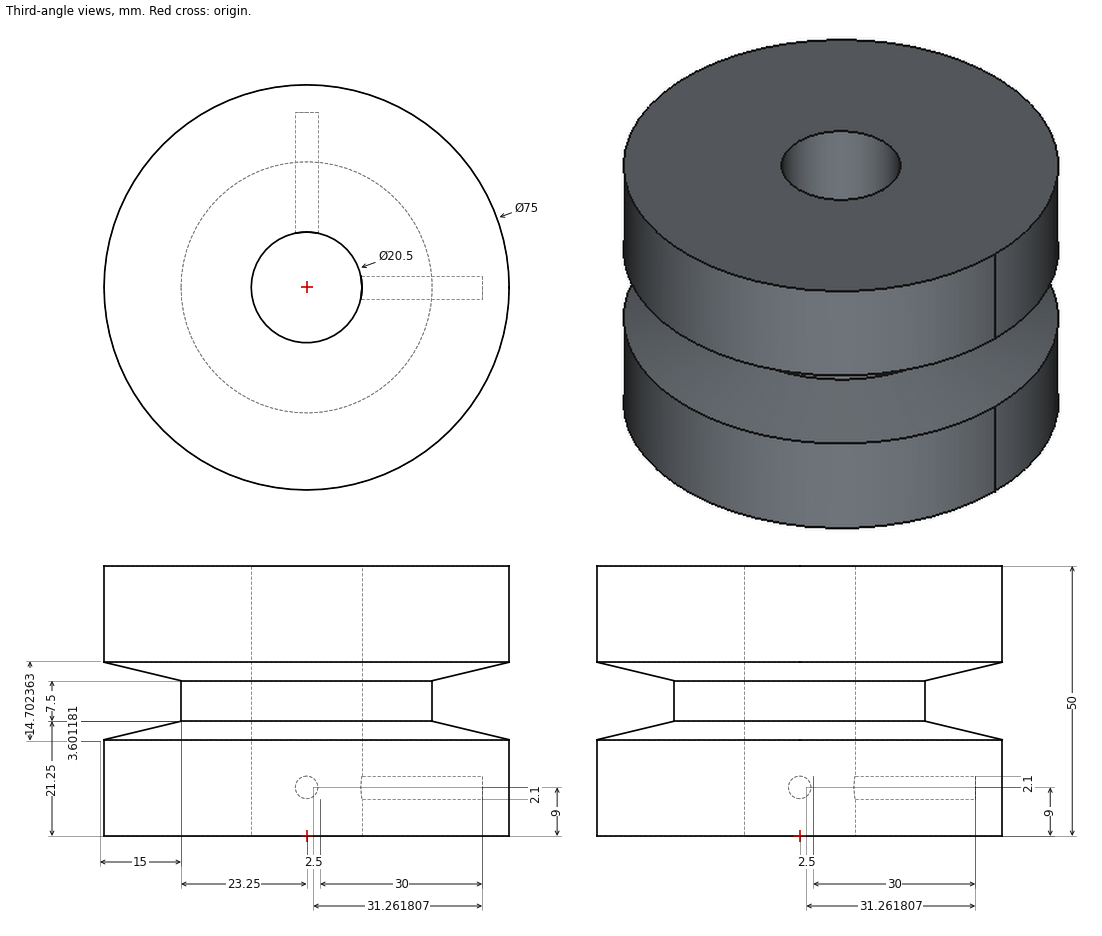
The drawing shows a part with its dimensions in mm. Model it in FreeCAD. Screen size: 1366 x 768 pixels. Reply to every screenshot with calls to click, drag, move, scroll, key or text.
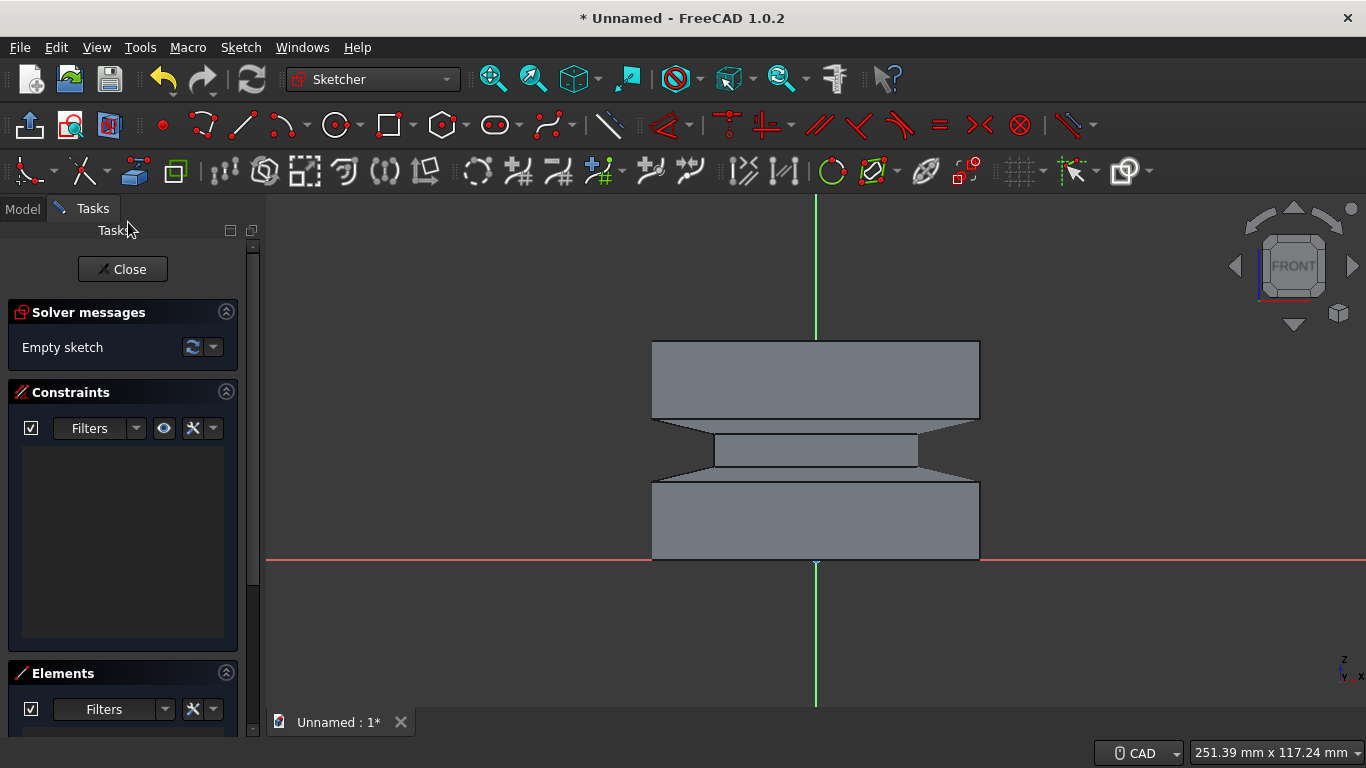
key(q)
key(s)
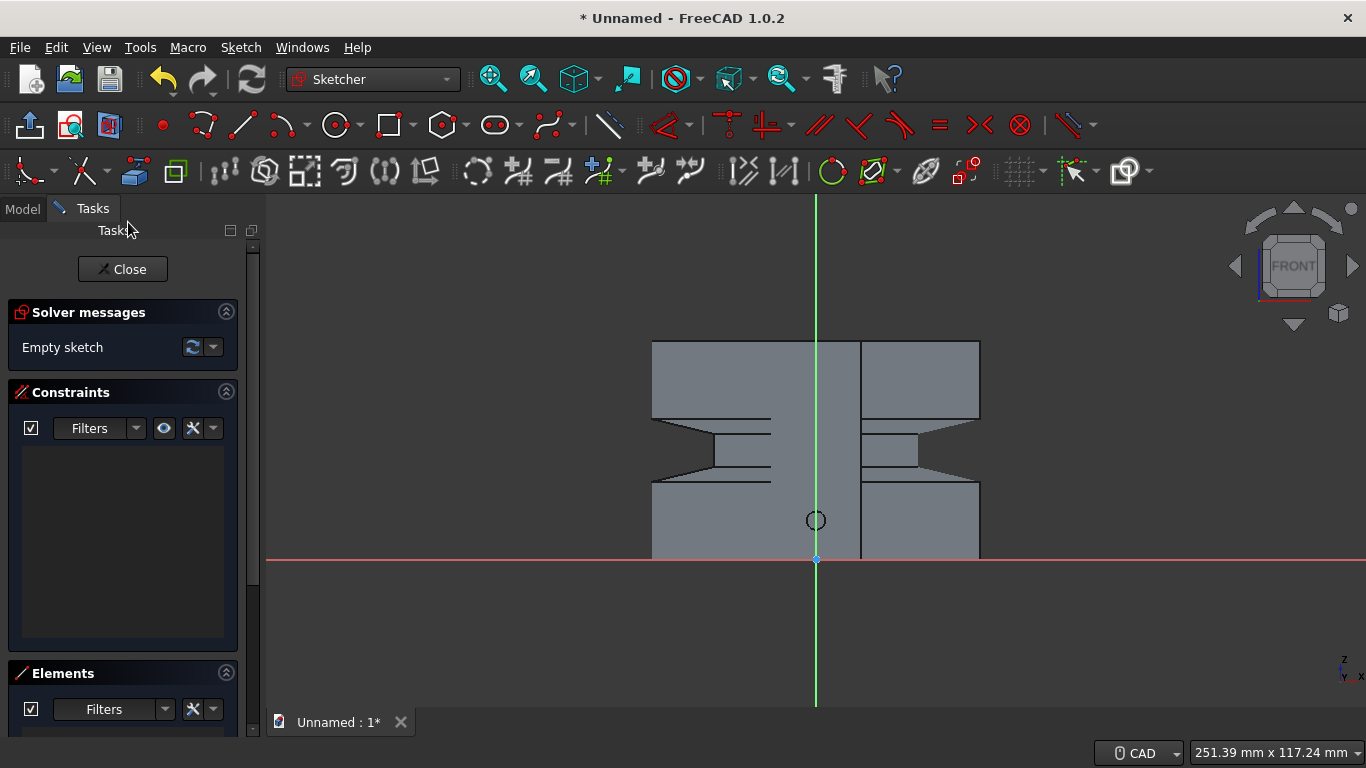
scroll(912, 579, up, 6)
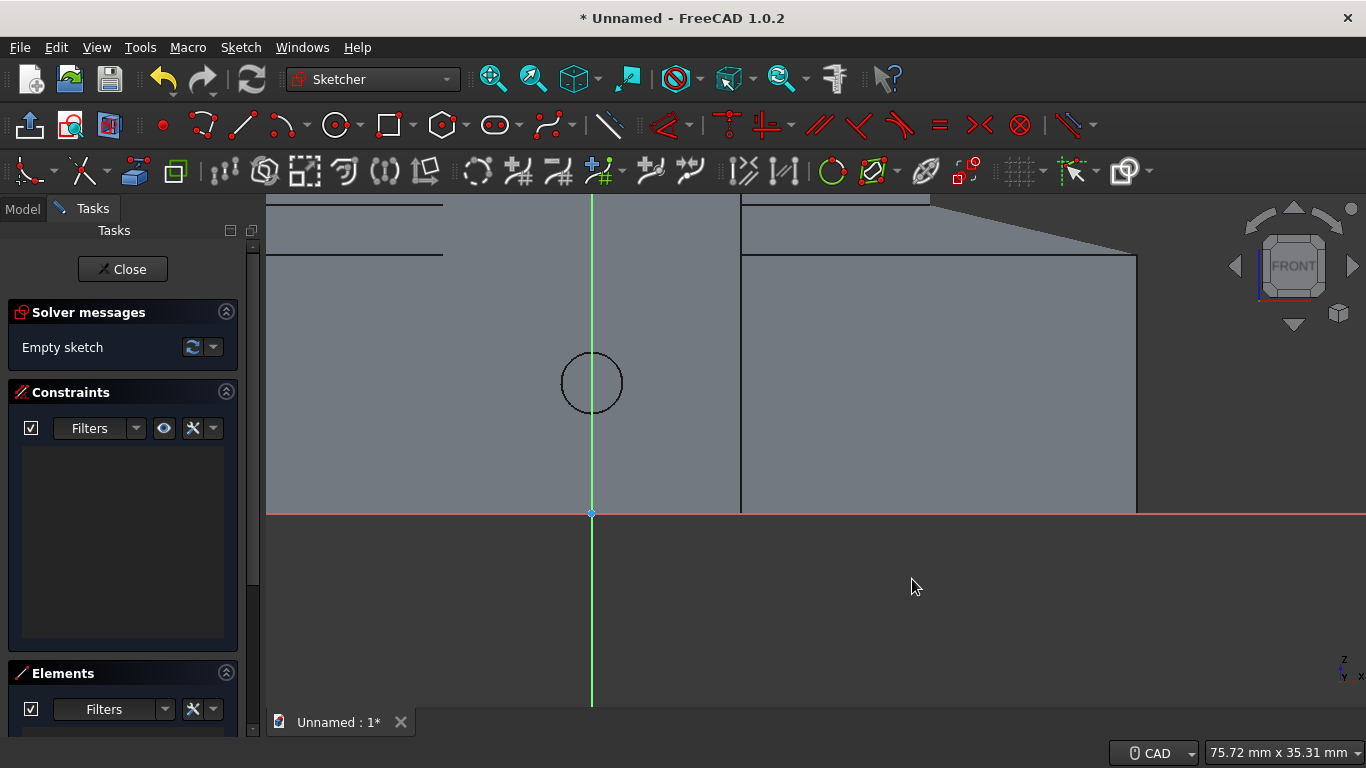
key(g)
key(m)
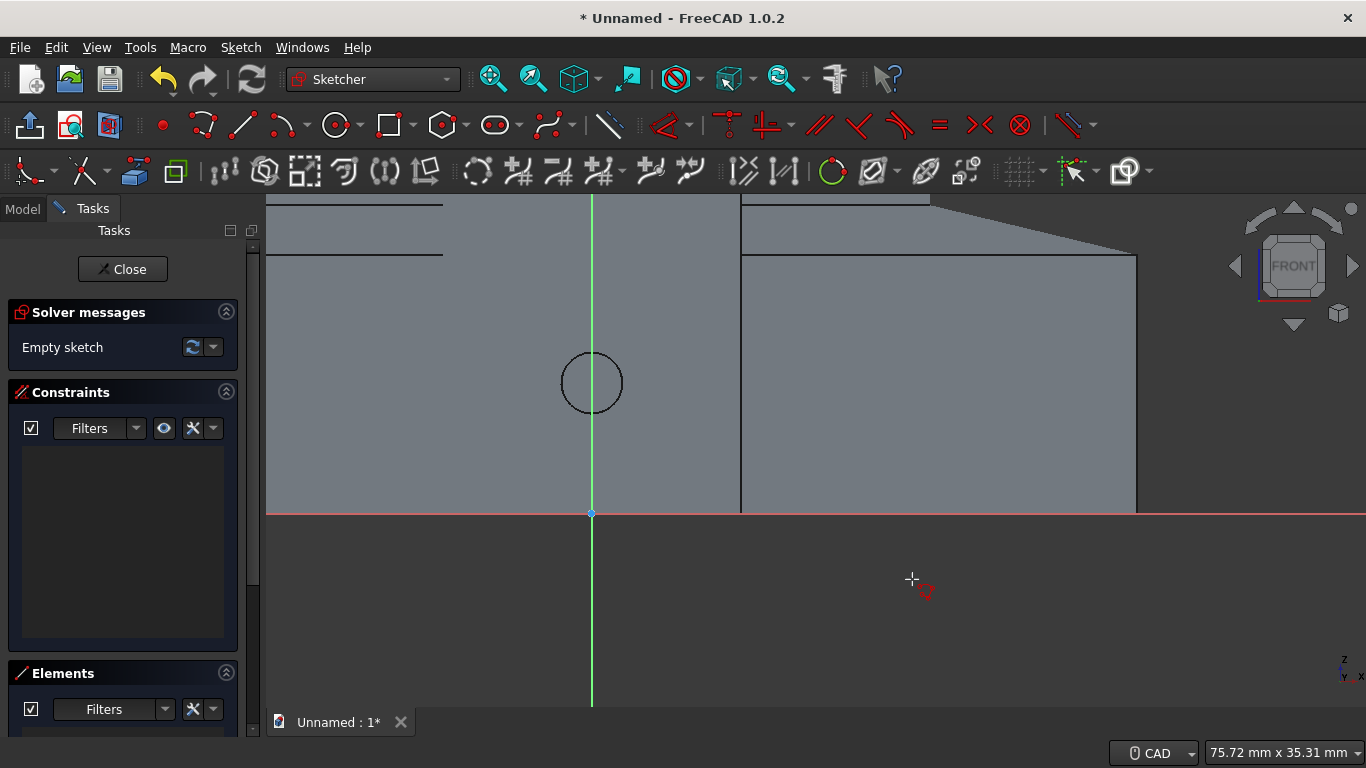
click(628, 414)
click(610, 383)
click(1064, 383)
click(1064, 414)
click(628, 415)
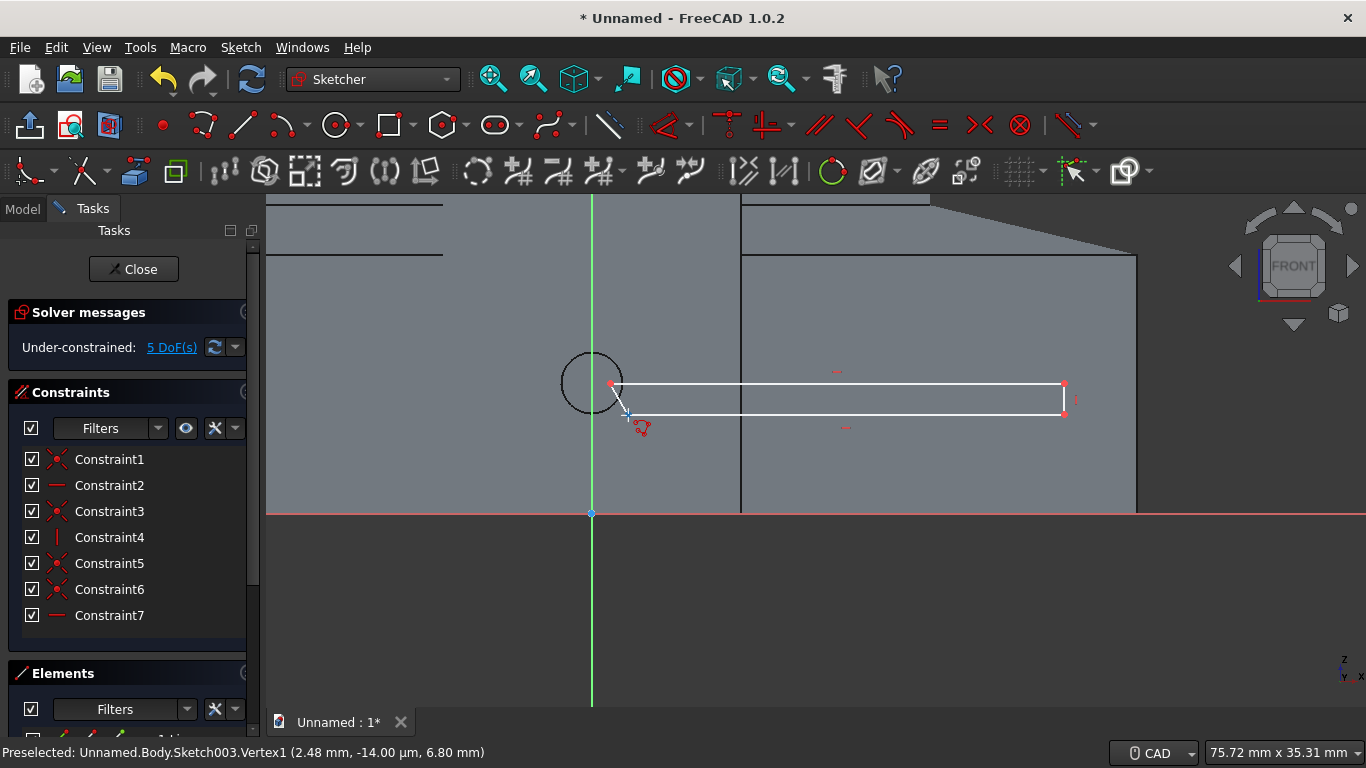
click(244, 126)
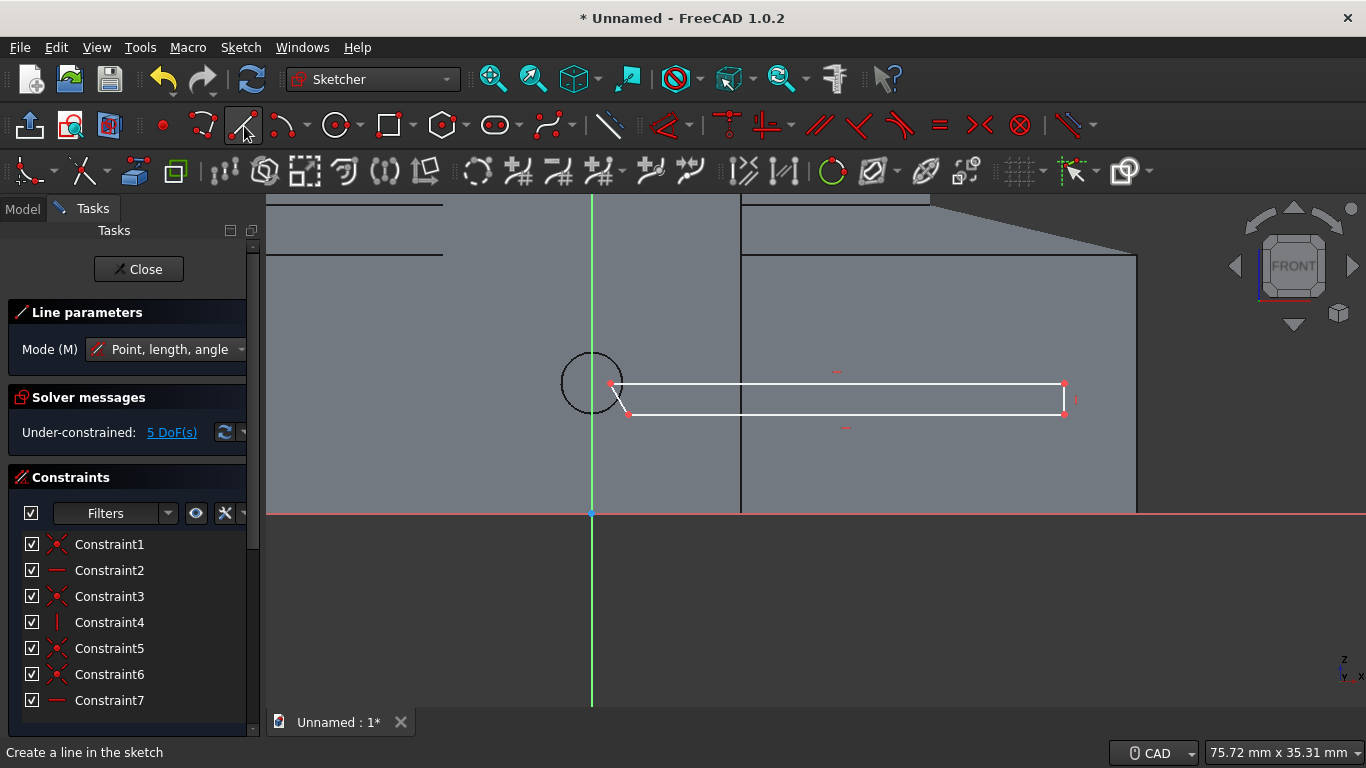
click(564, 383)
click(428, 383)
key(Escape)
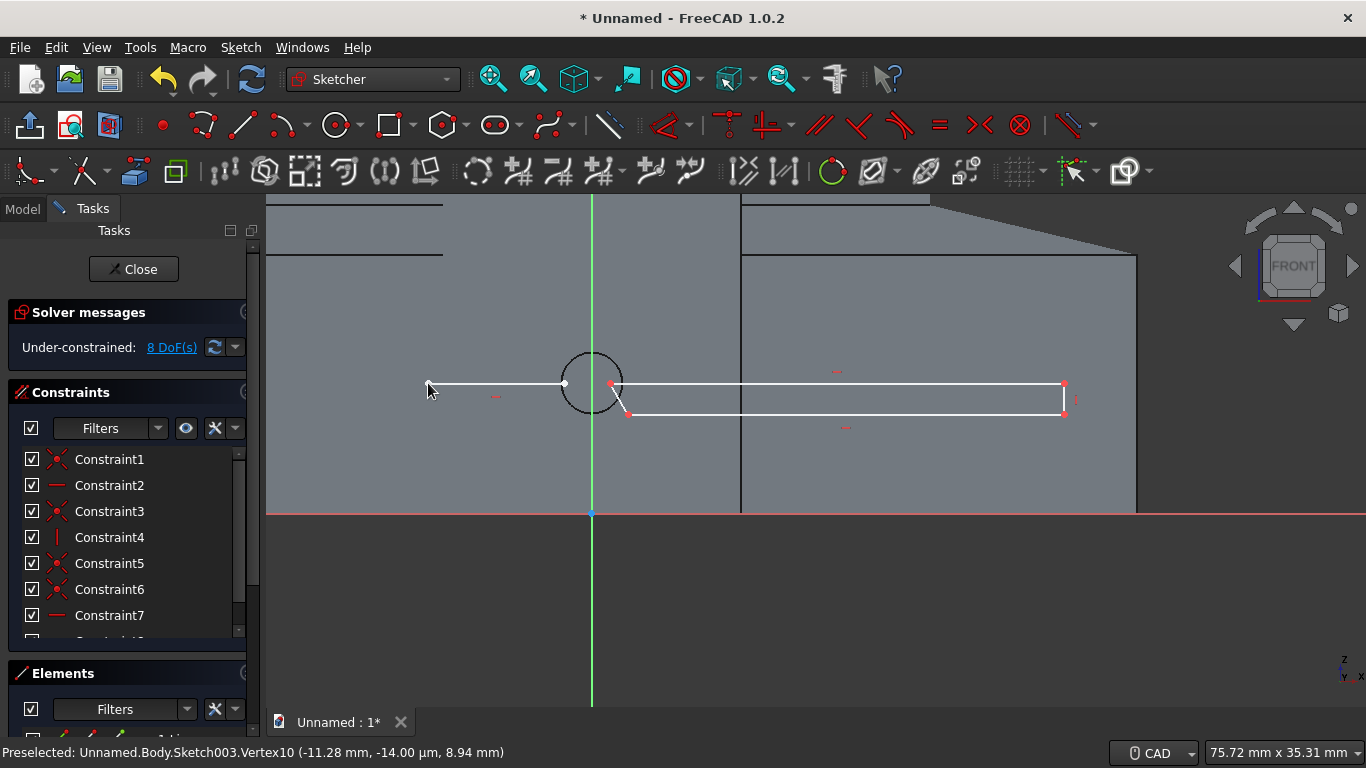
click(523, 384)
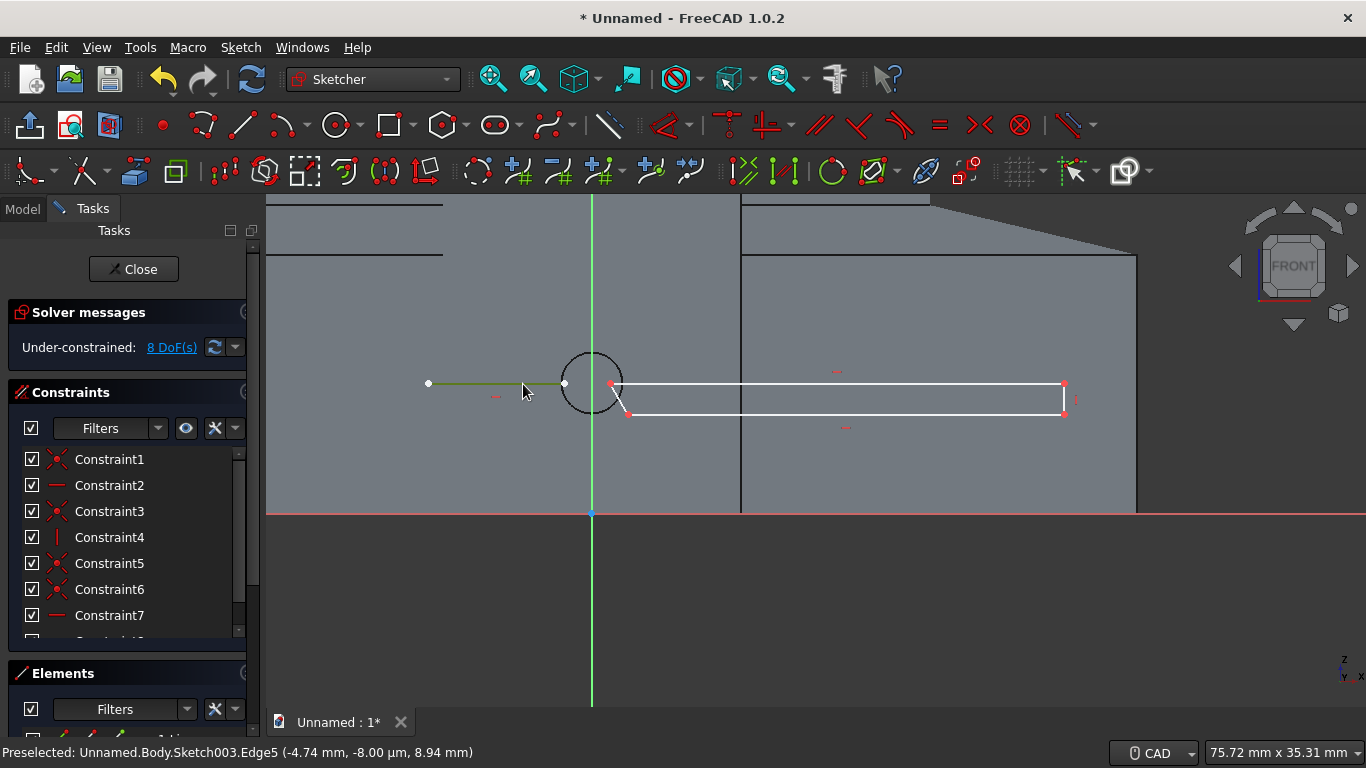
click(610, 126)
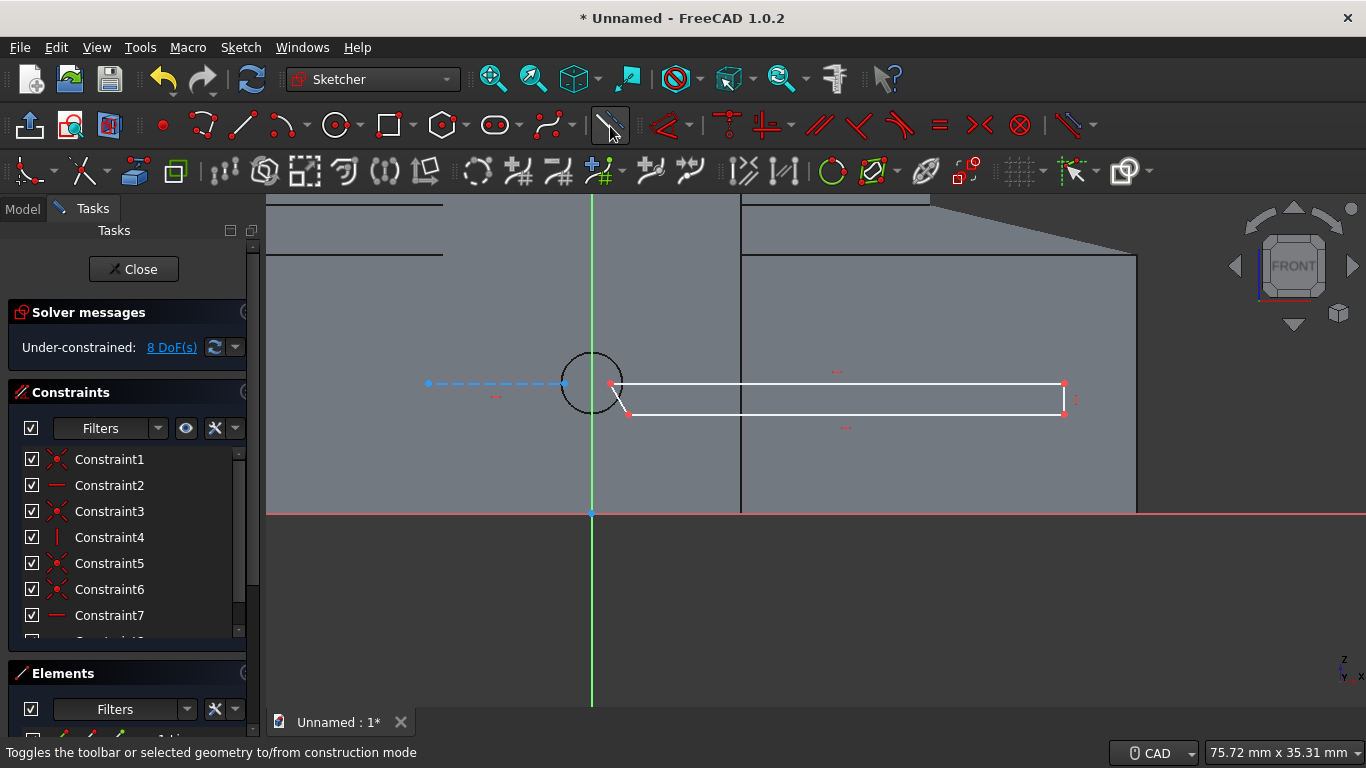
key(d)